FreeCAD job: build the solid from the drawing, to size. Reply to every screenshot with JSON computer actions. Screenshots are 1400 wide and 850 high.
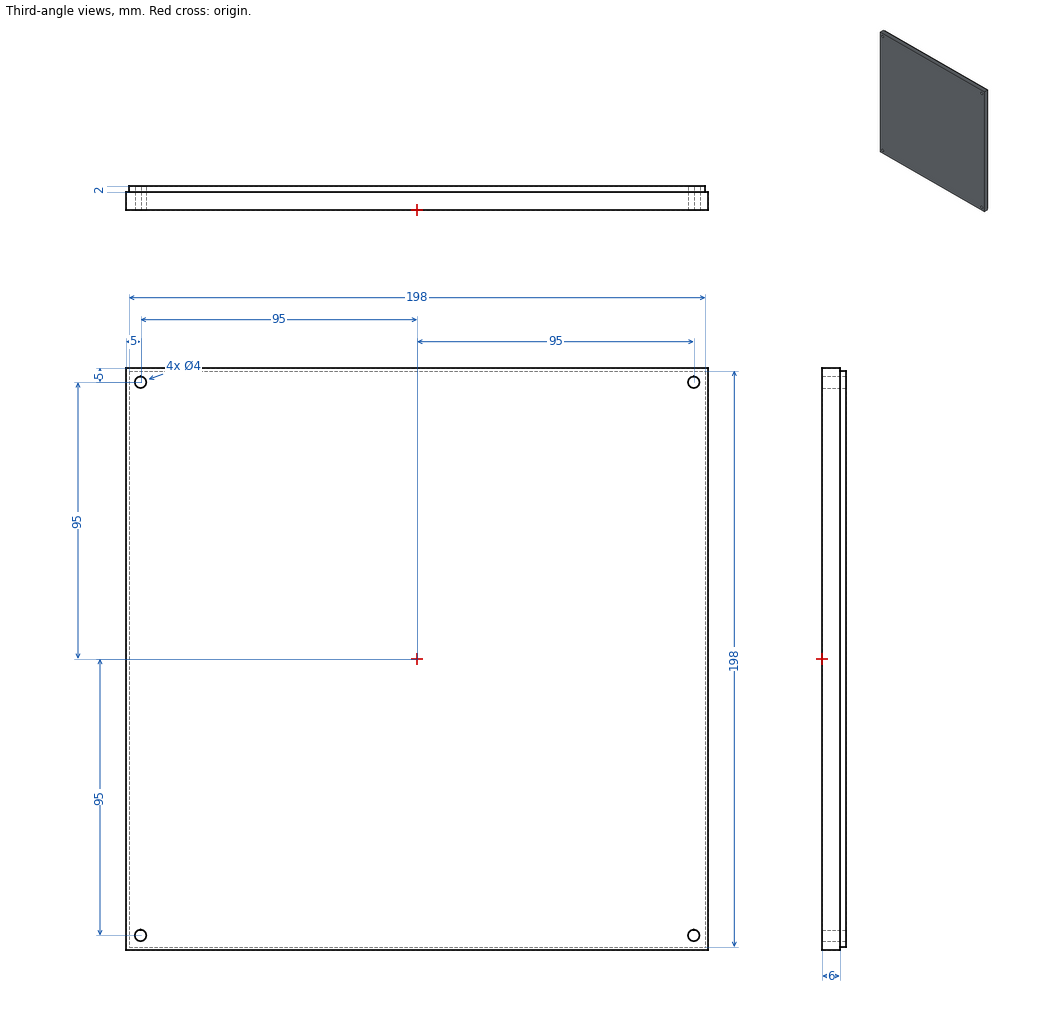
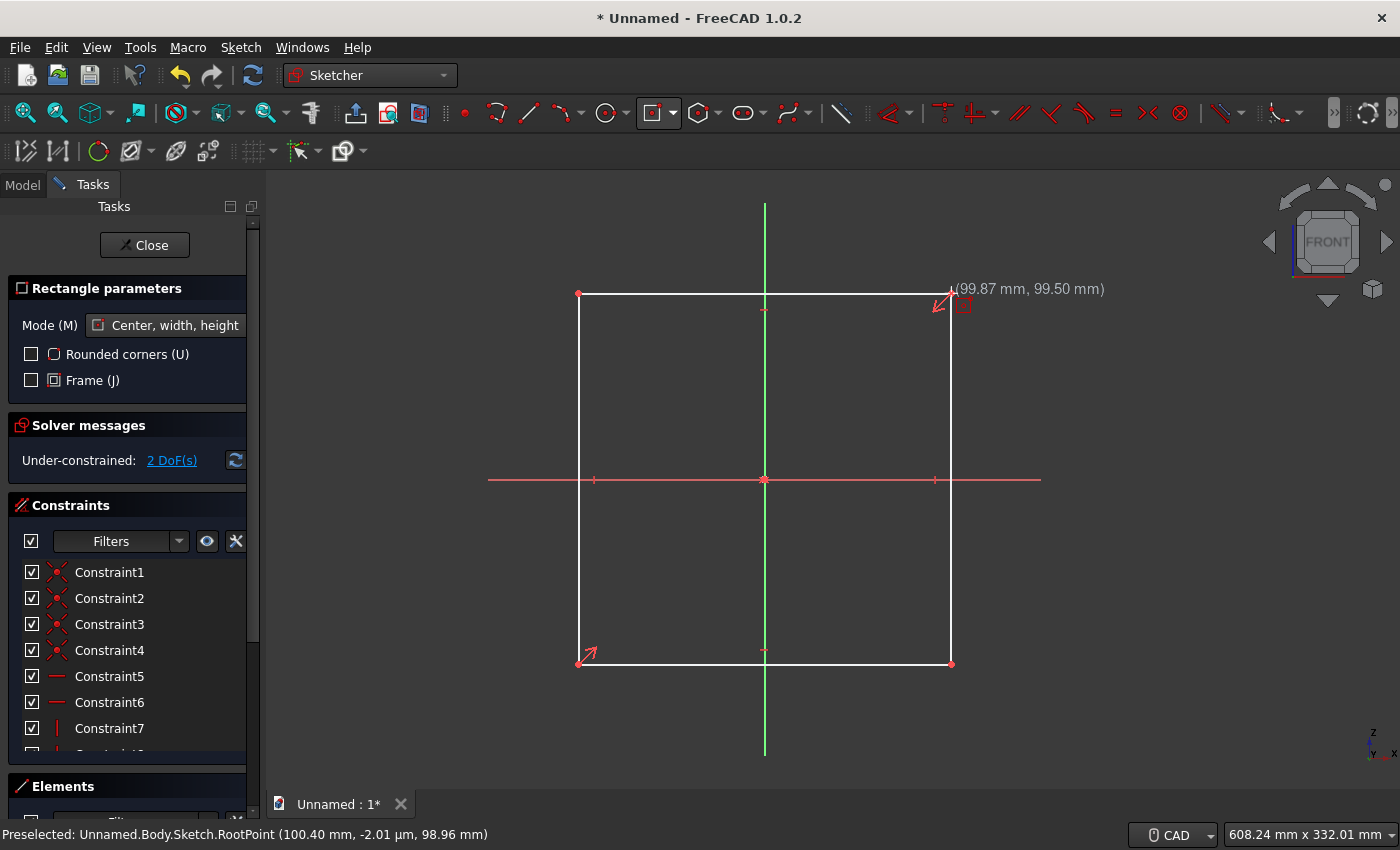
{"action": "left_click", "coordinate": [606, 114]}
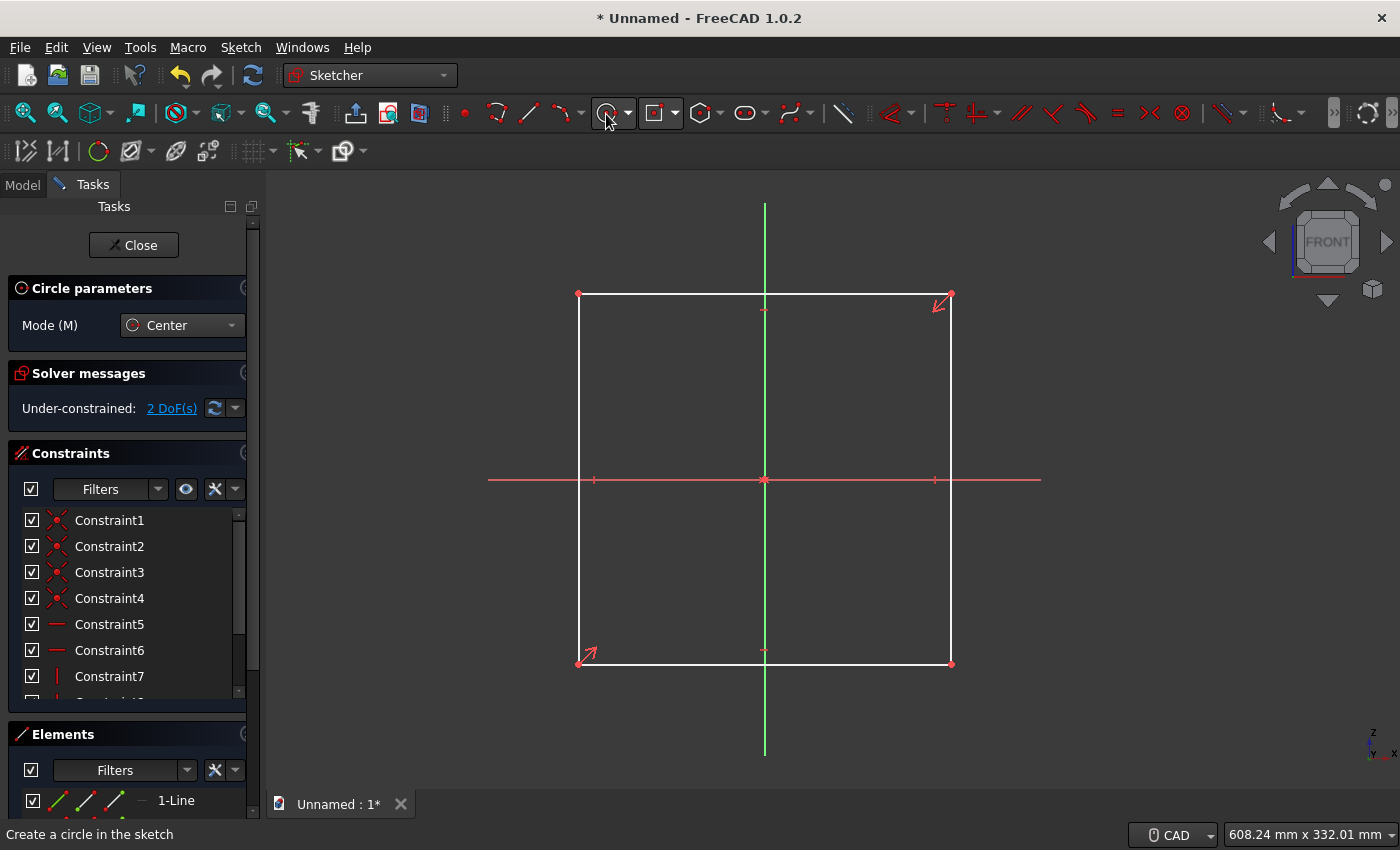
{"action": "scroll", "coordinate": [588, 302], "scroll_direction": "up", "scroll_amount": 10}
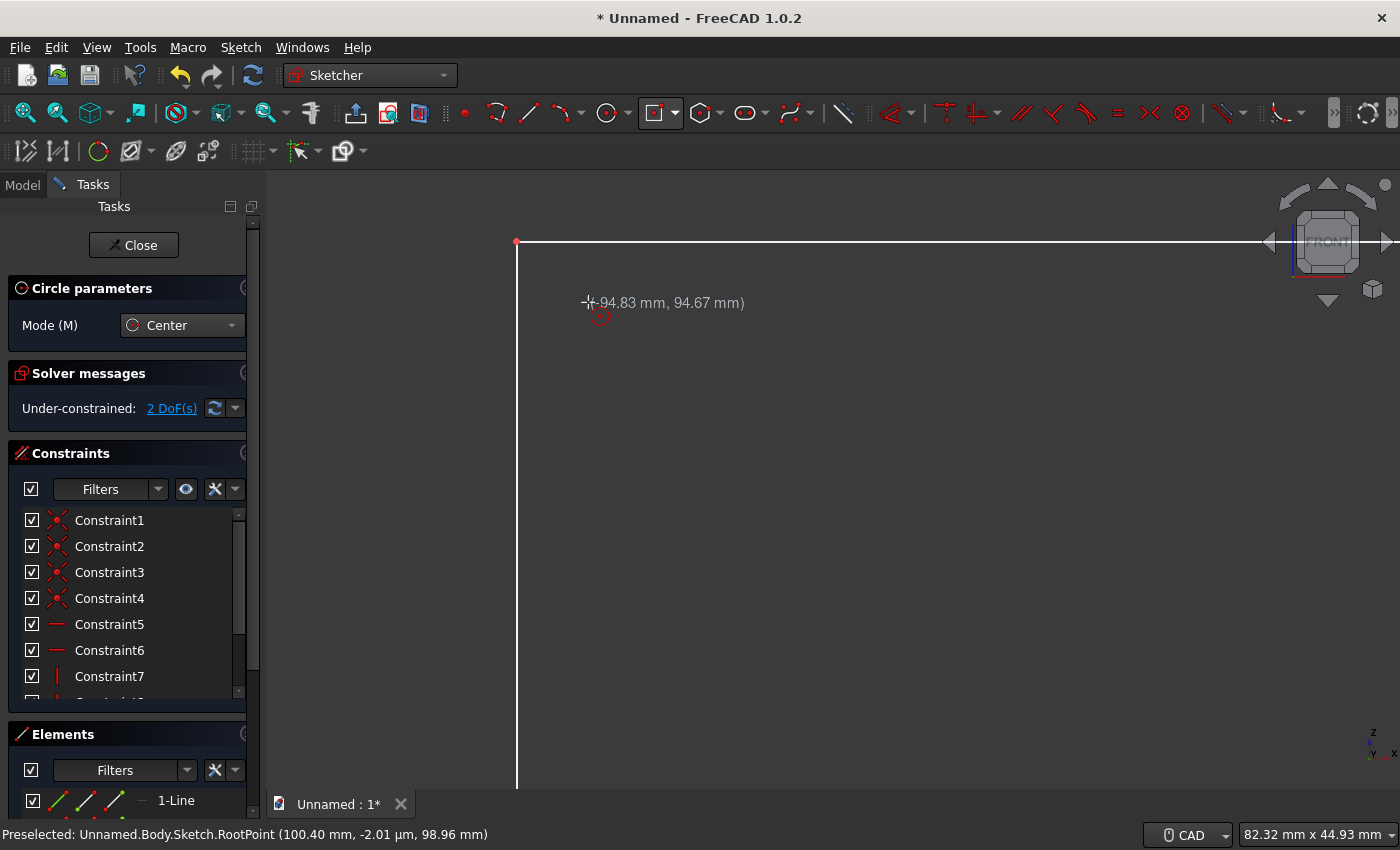
{"action": "scroll", "coordinate": [588, 302], "scroll_direction": "down", "scroll_amount": 10}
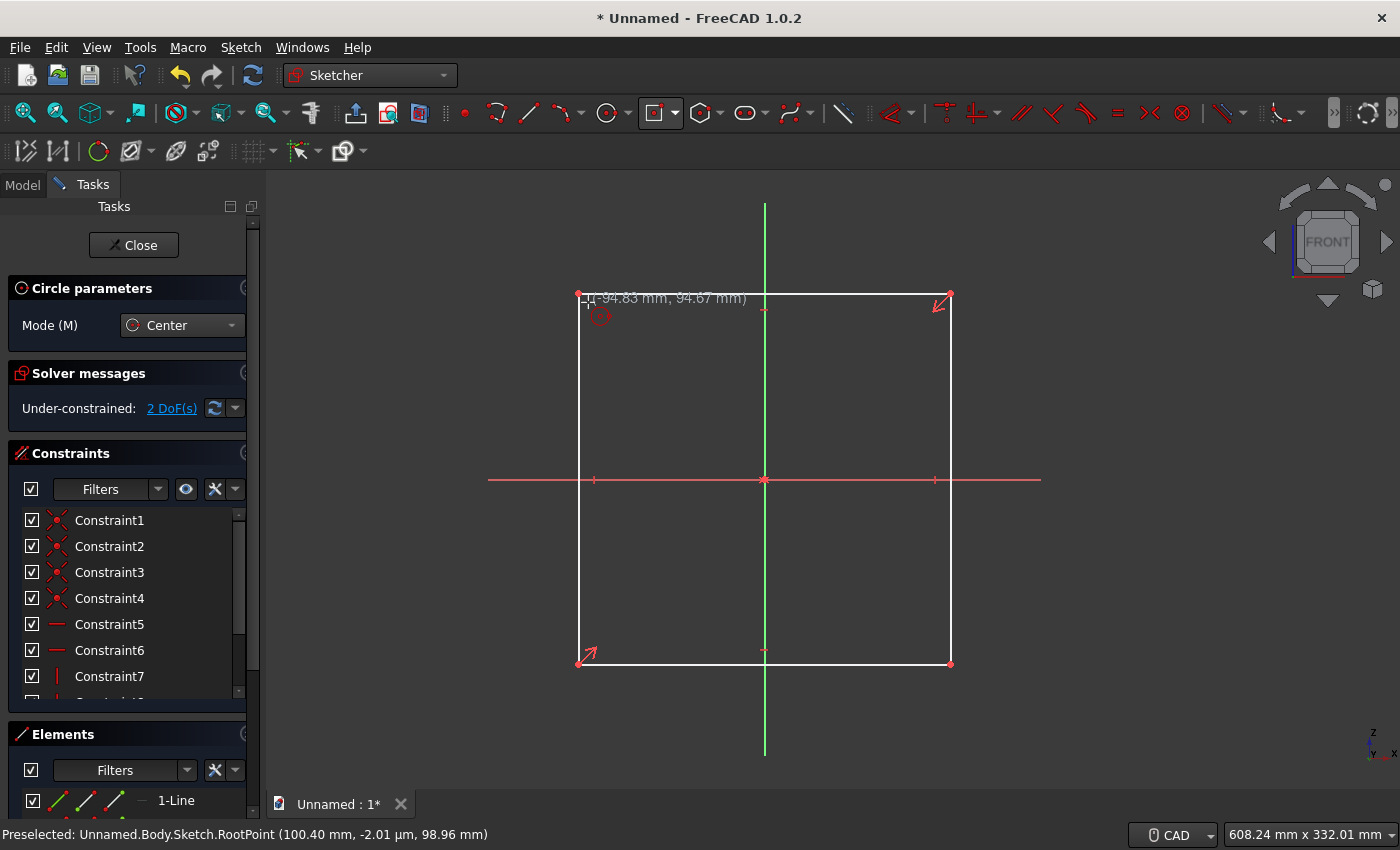
{"action": "scroll", "coordinate": [588, 302], "scroll_direction": "up", "scroll_amount": 3}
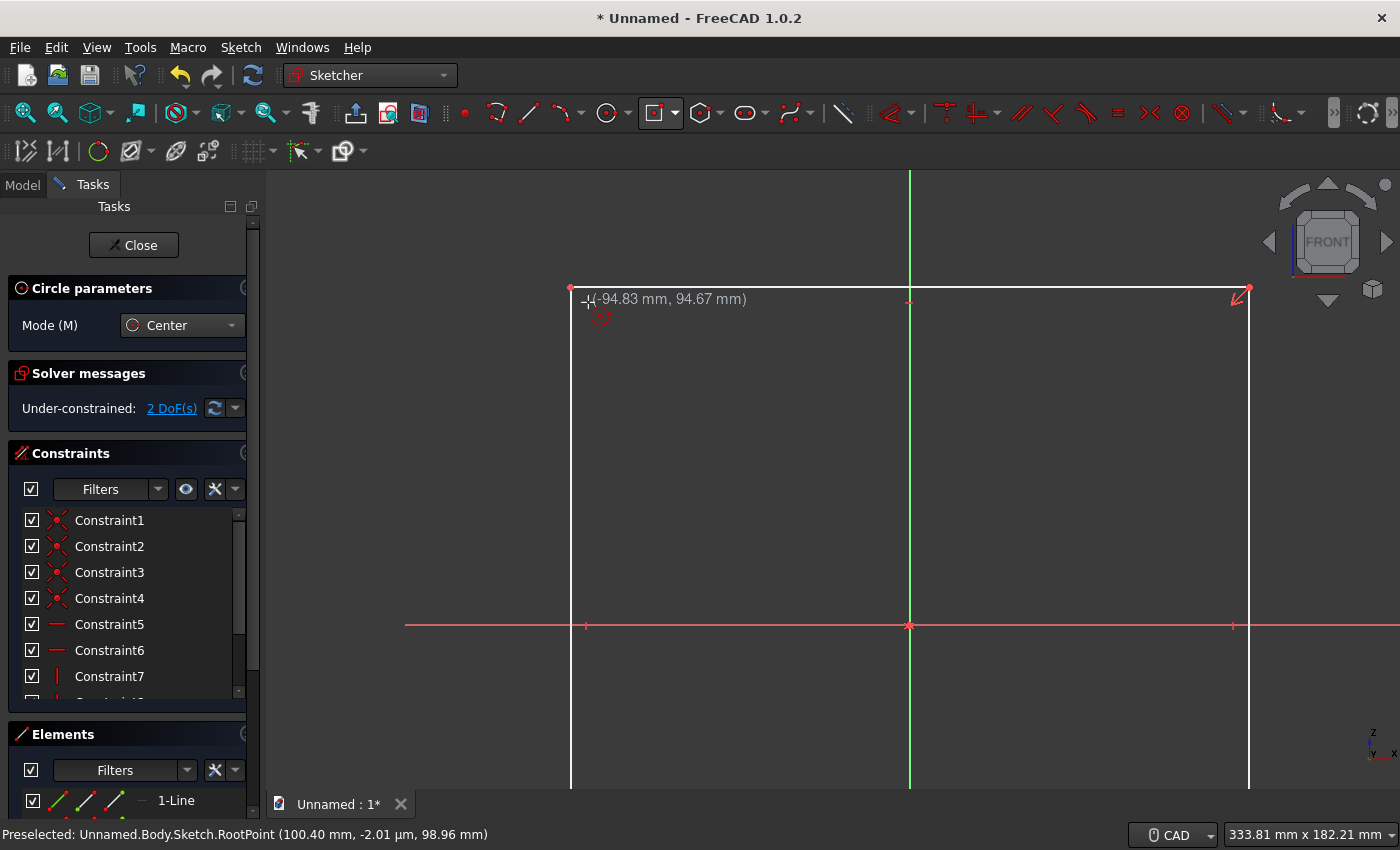
{"action": "left_click", "coordinate": [587, 303]}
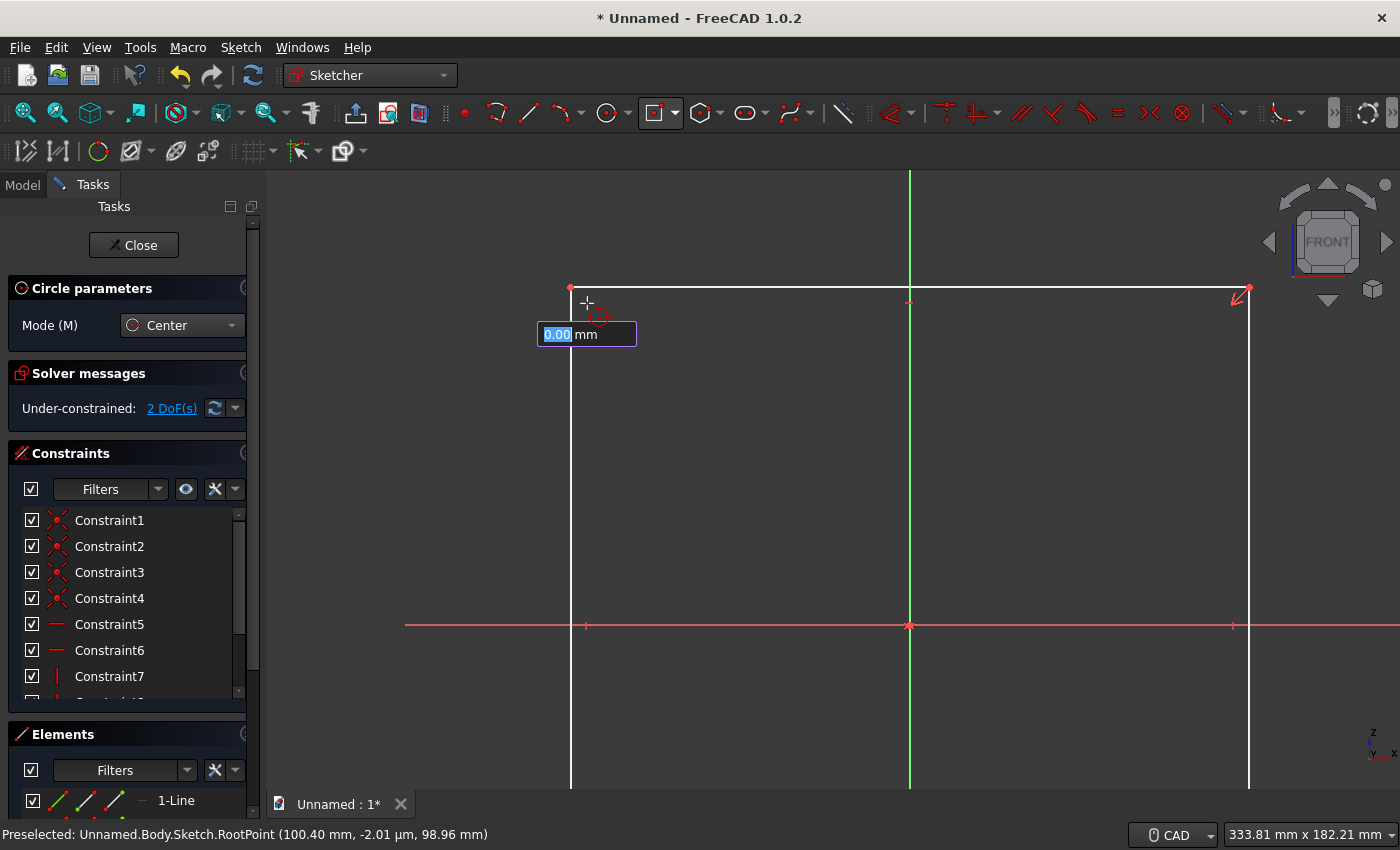
{"action": "scroll", "coordinate": [592, 307], "scroll_direction": "up", "scroll_amount": 5}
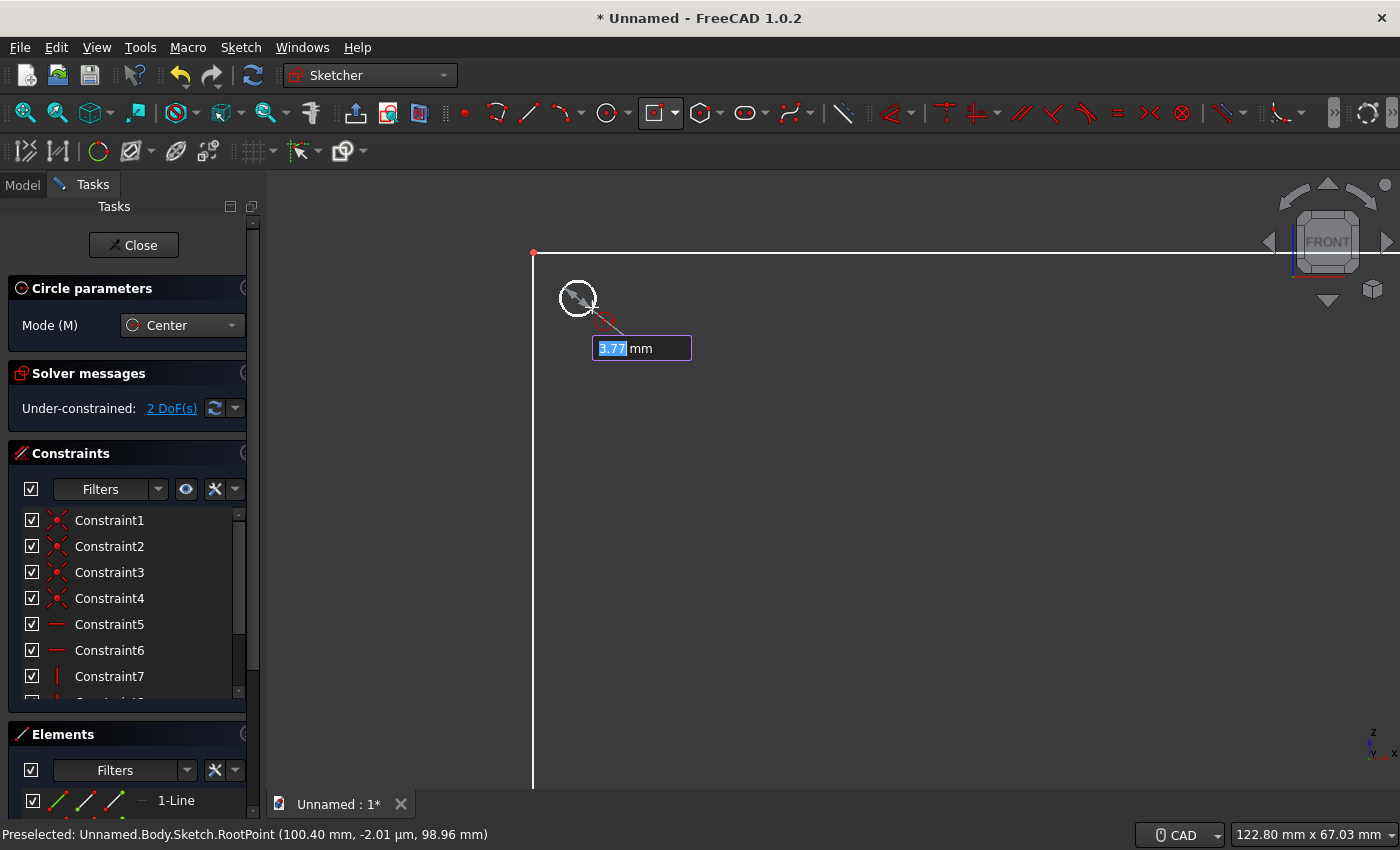
{"action": "left_click", "coordinate": [592, 308]}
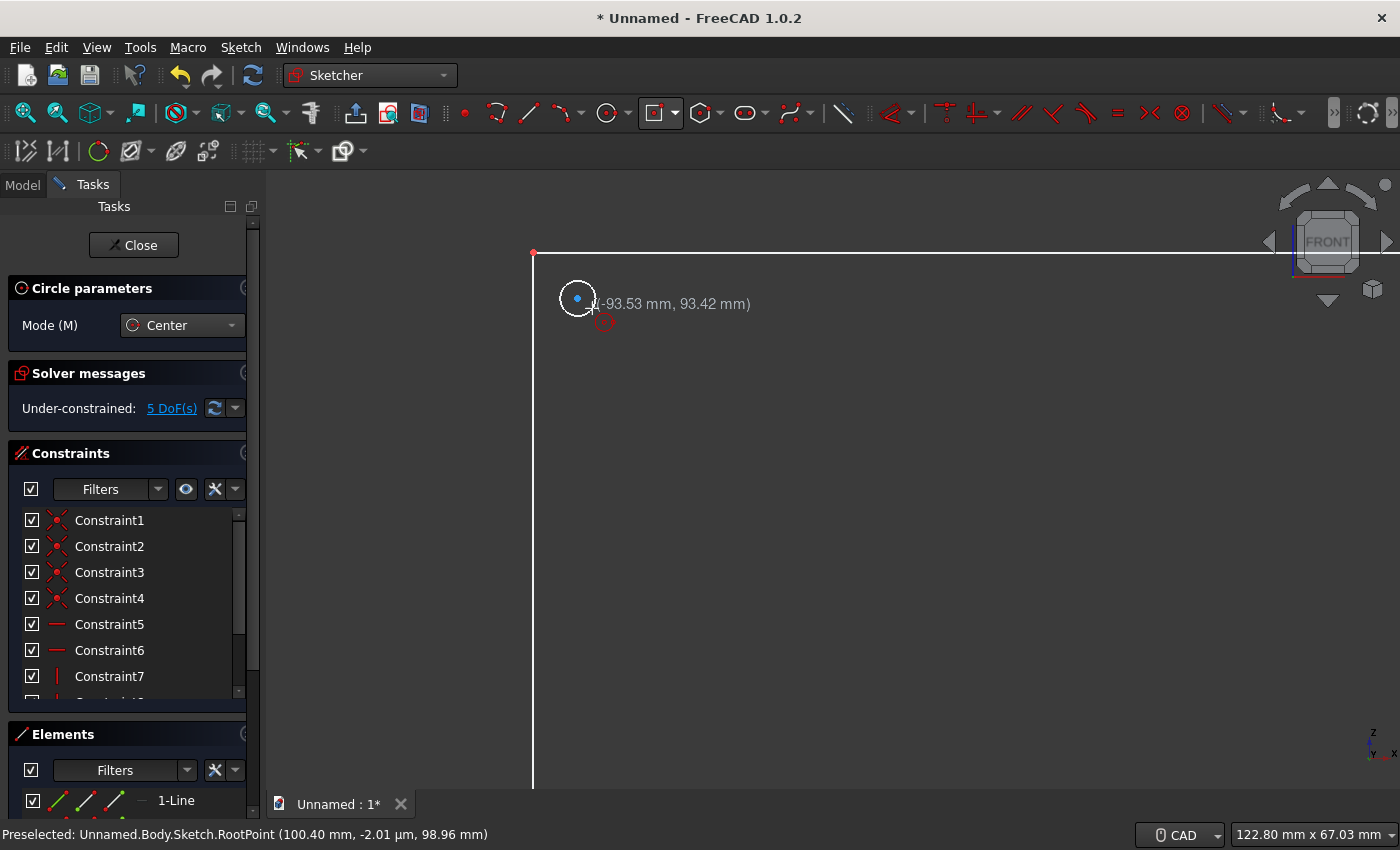
{"action": "scroll", "coordinate": [590, 304], "scroll_direction": "down", "scroll_amount": 8}